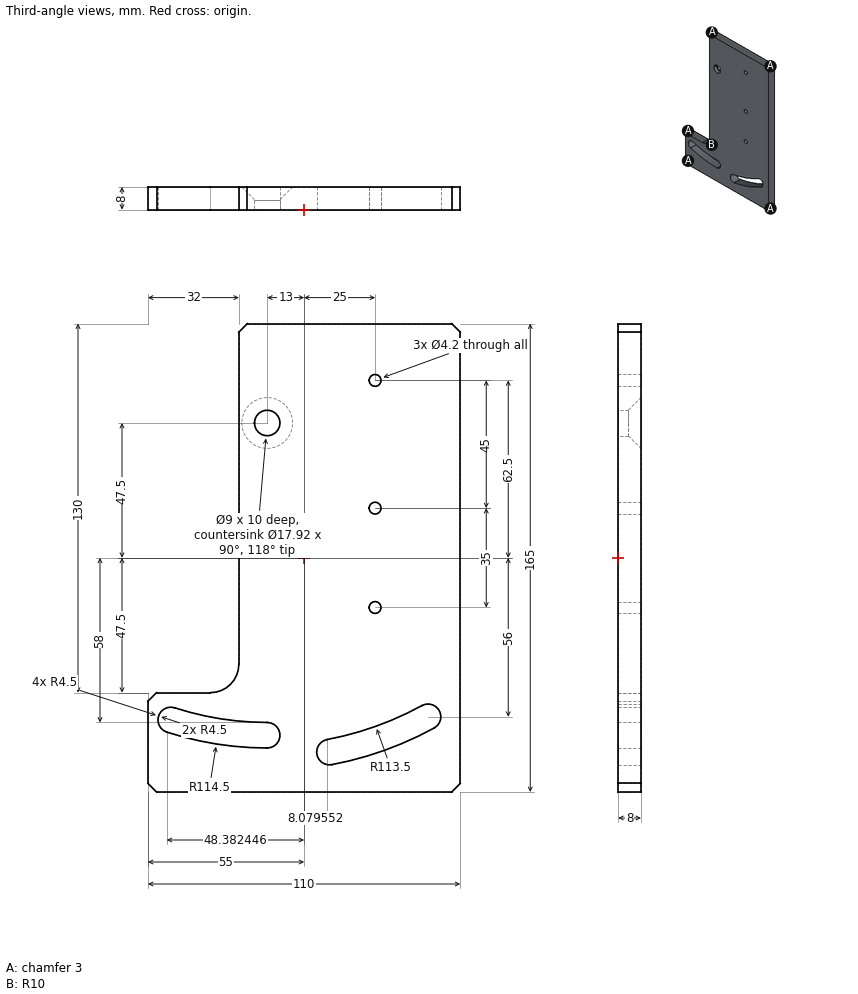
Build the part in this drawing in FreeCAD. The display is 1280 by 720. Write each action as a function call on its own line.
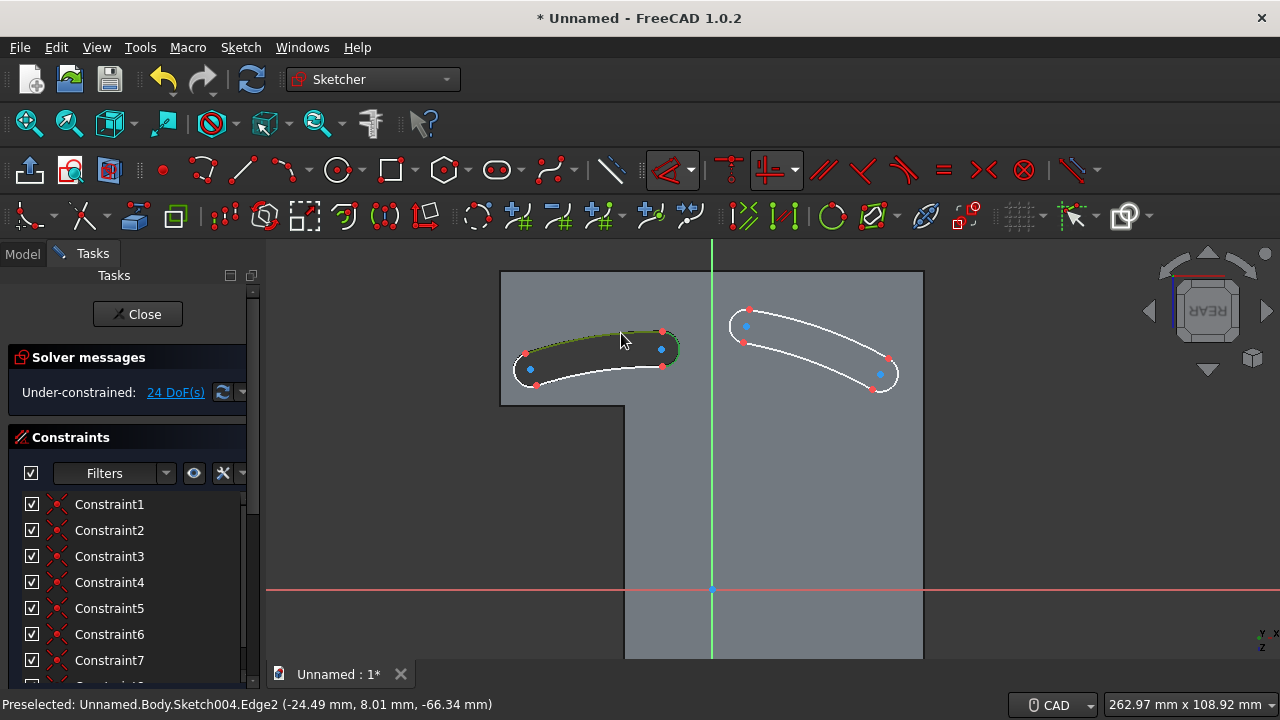
click(904, 170)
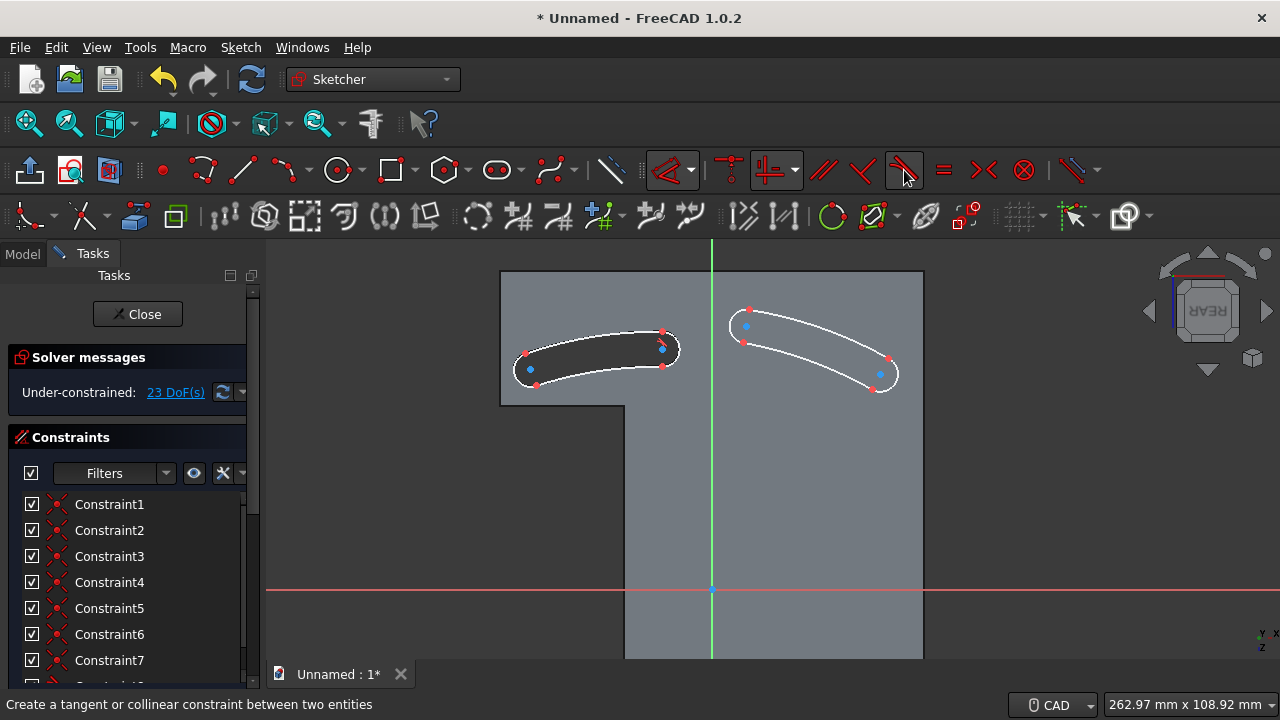
click(676, 360)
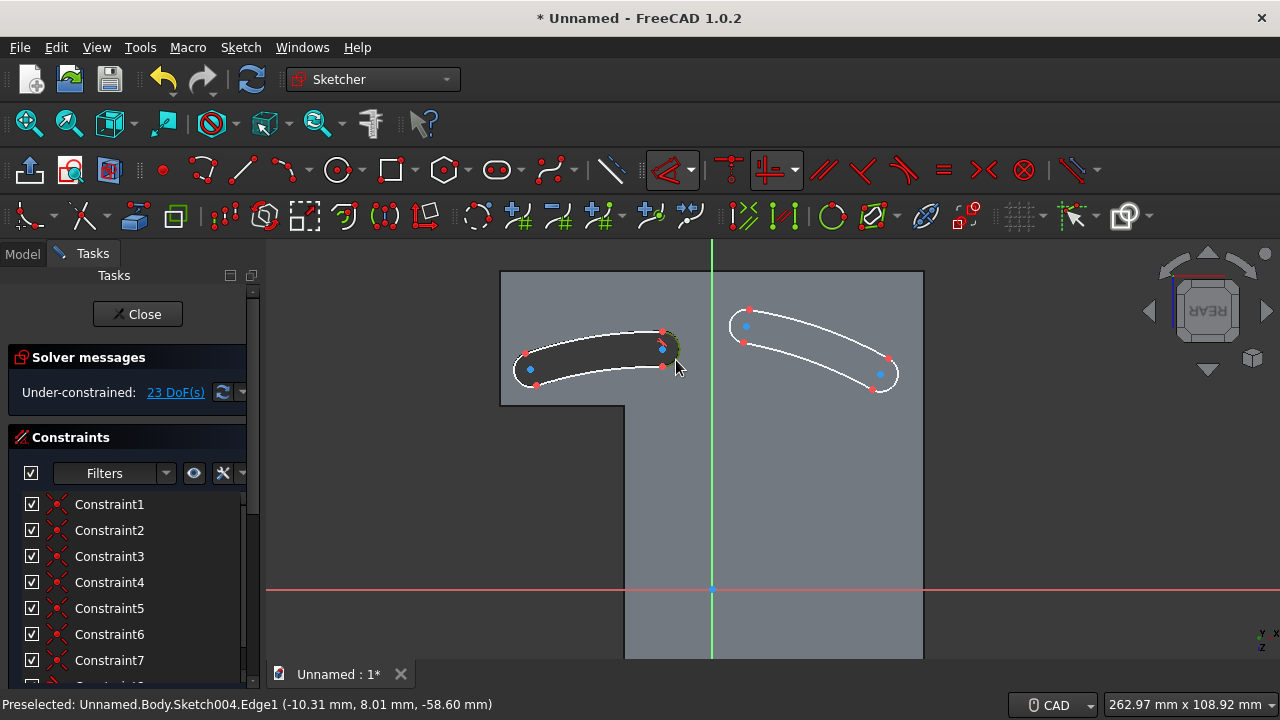
click(624, 368)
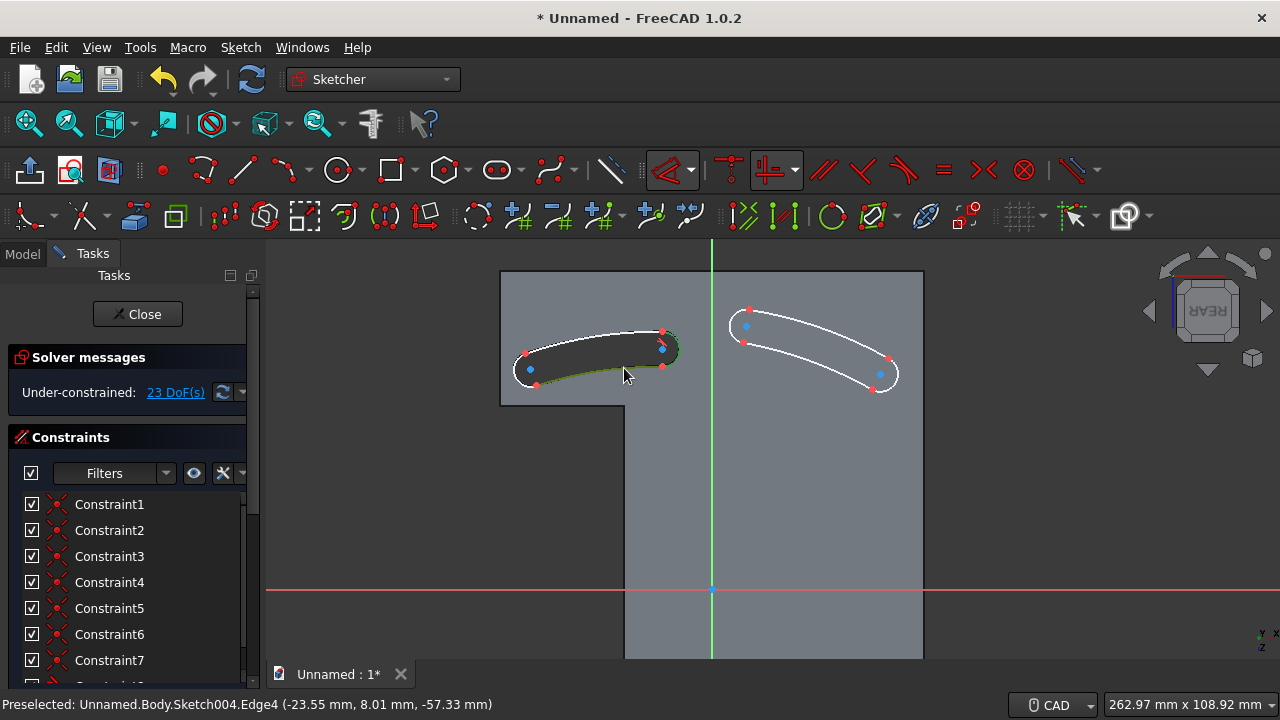
click(904, 170)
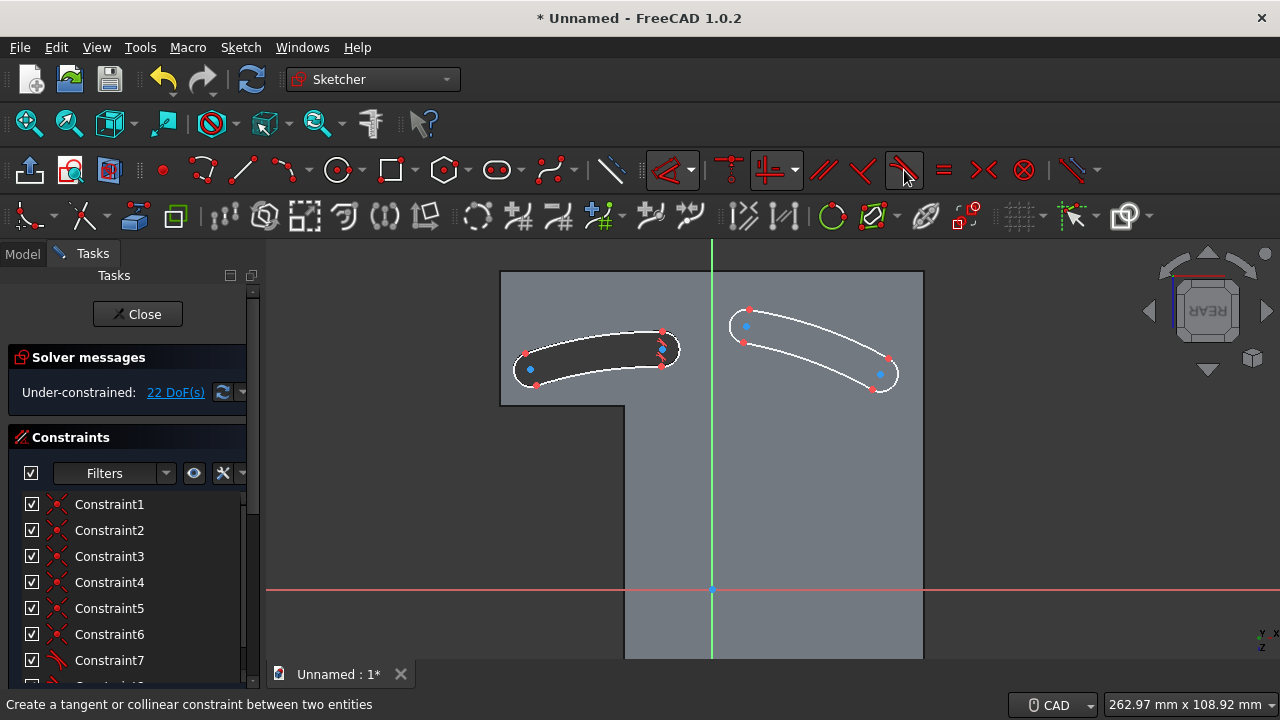
click(621, 333)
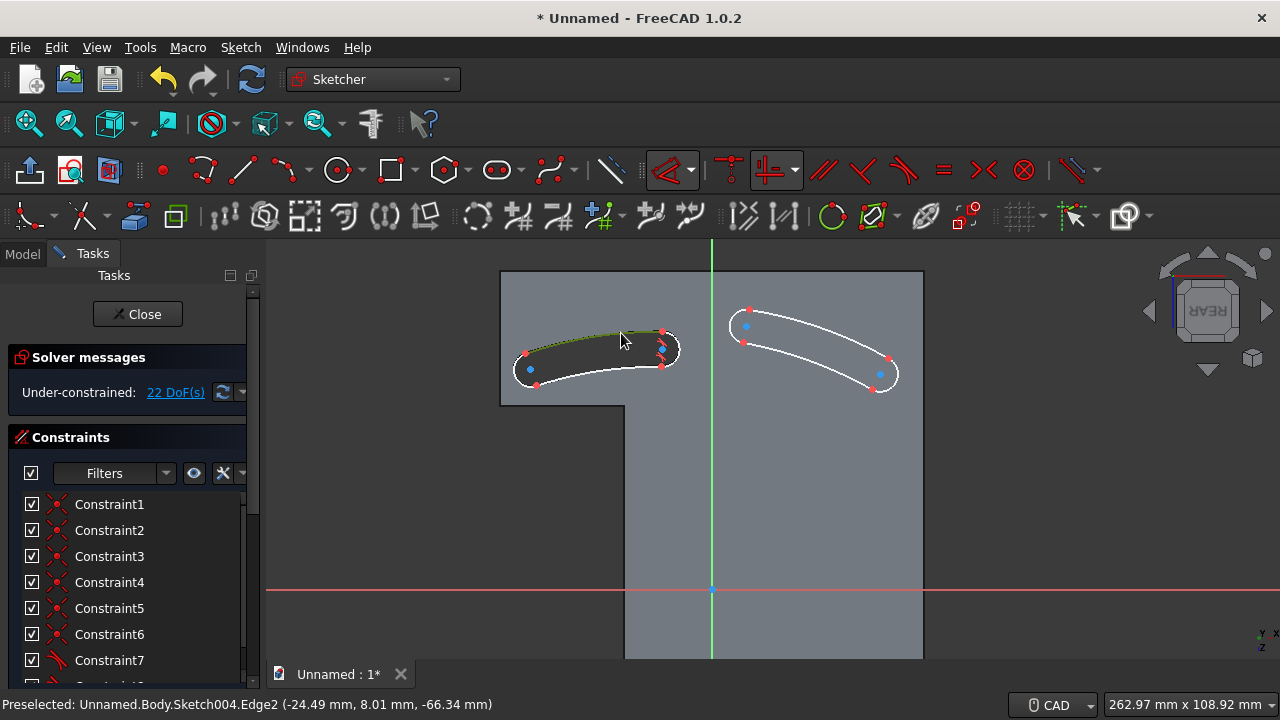
click(515, 365)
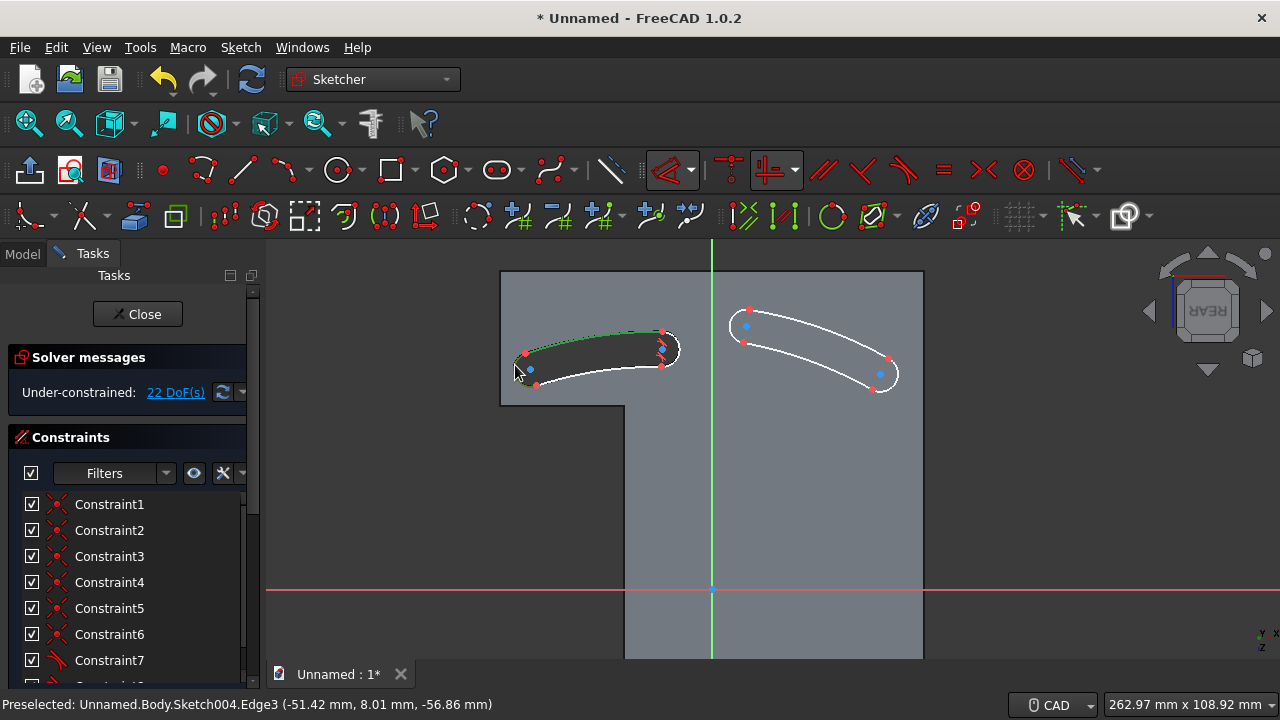
click(904, 170)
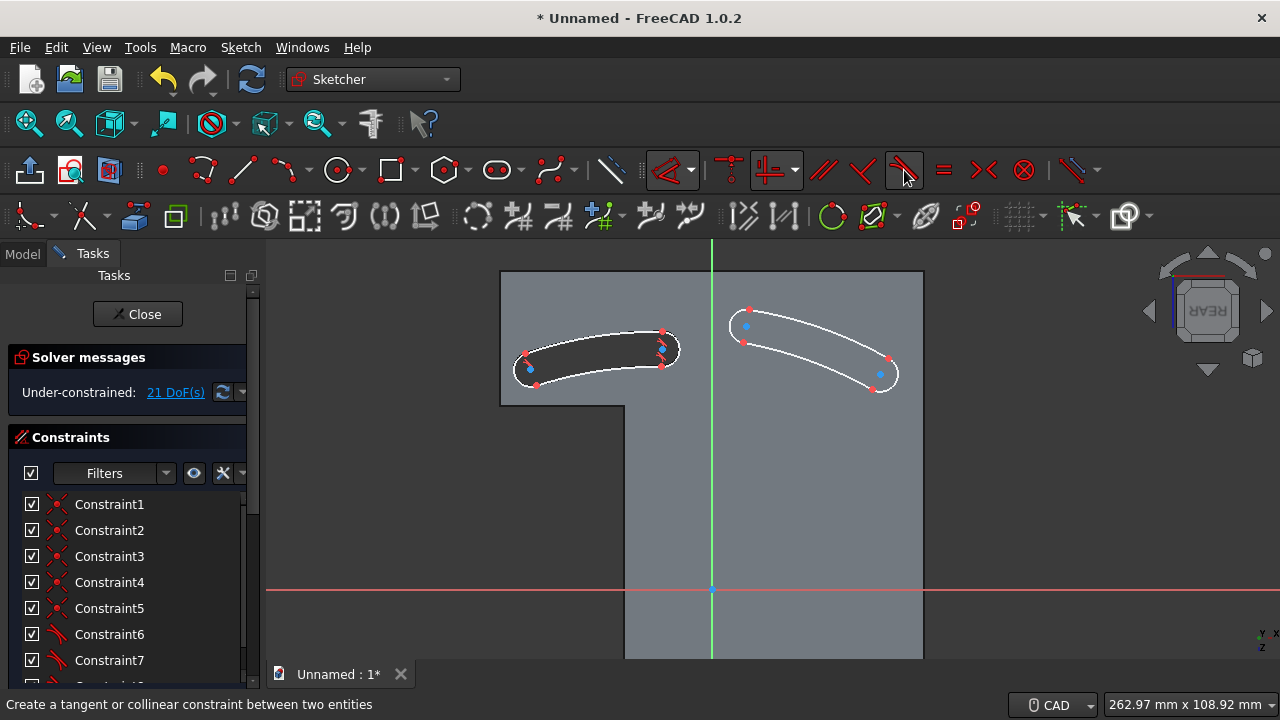
click(515, 365)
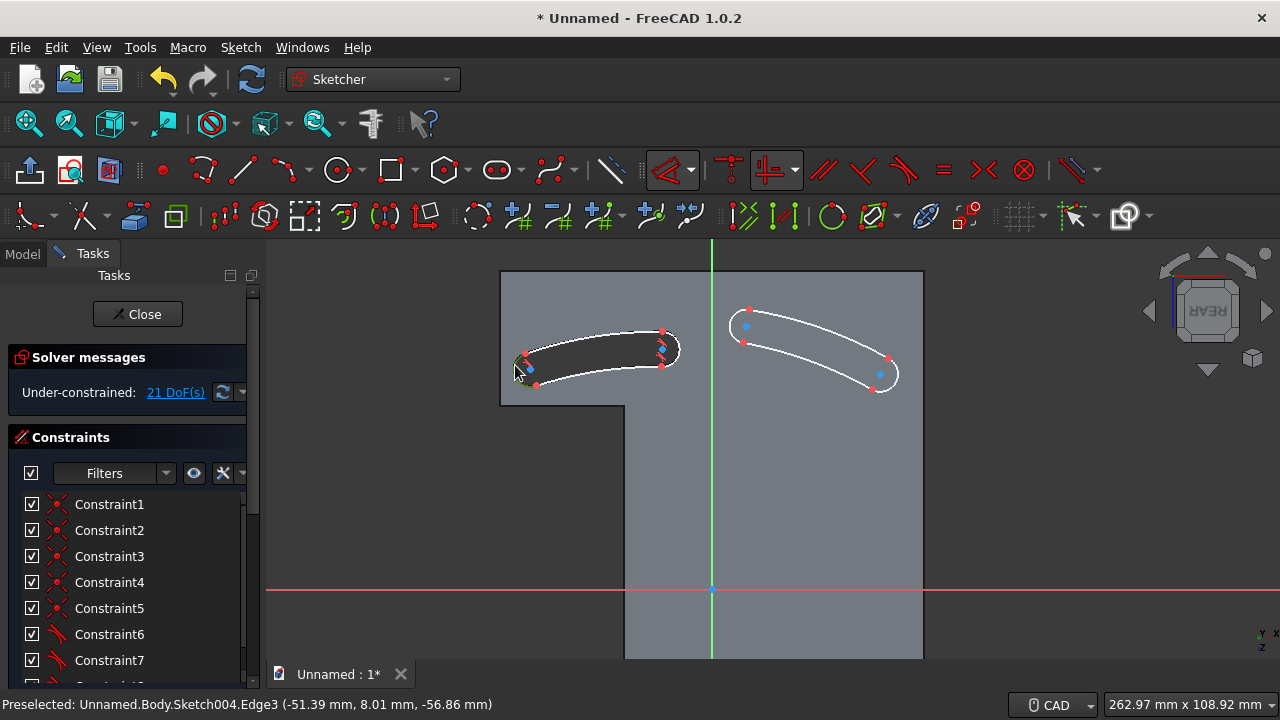
click(624, 368)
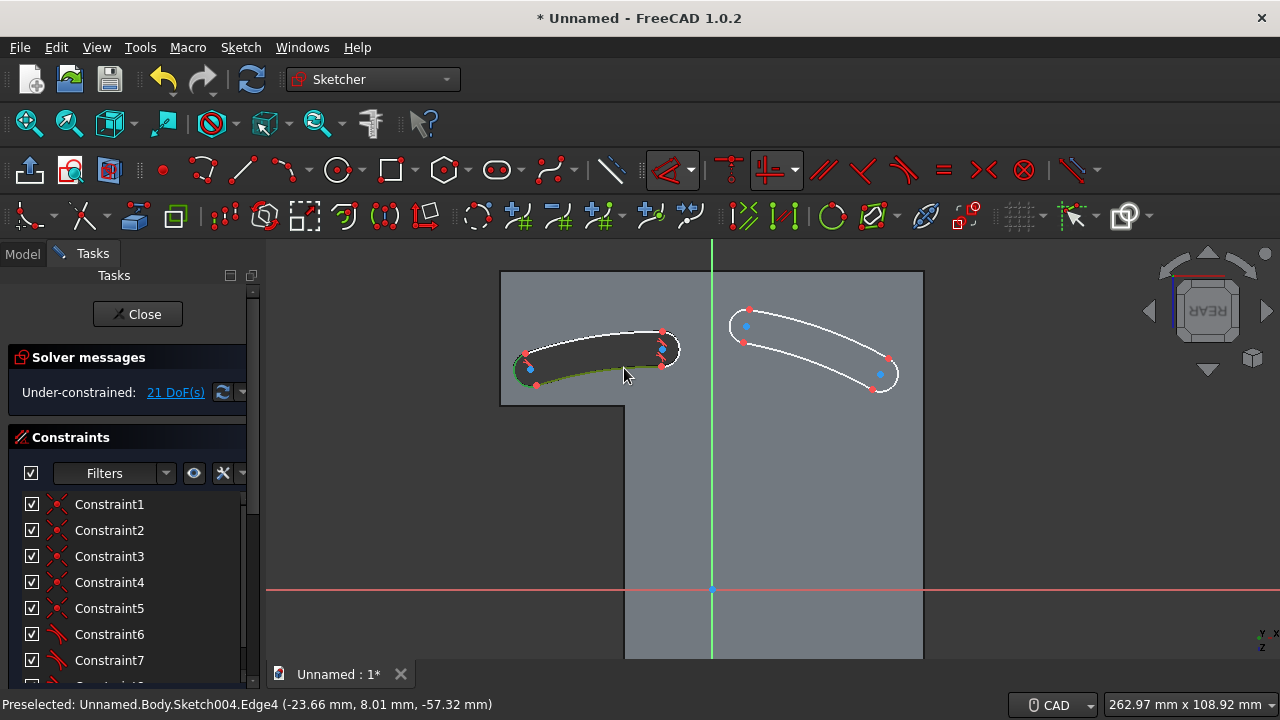
click(904, 170)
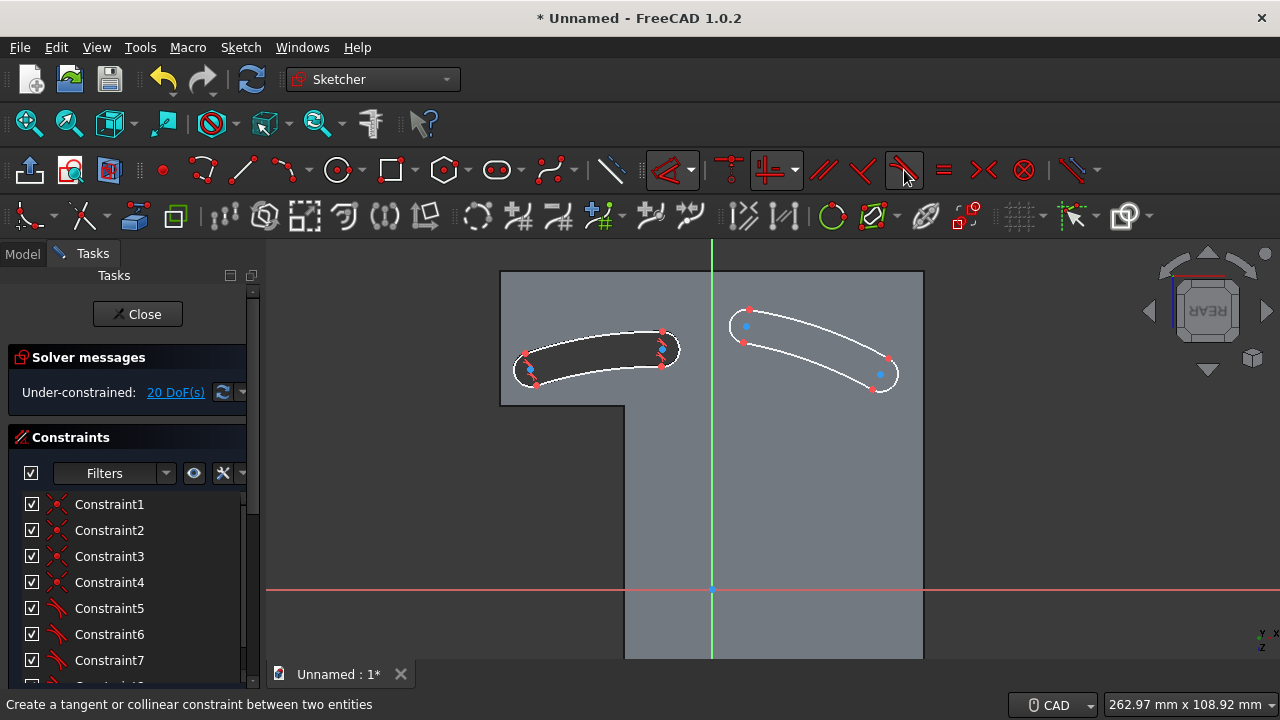
click(836, 371)